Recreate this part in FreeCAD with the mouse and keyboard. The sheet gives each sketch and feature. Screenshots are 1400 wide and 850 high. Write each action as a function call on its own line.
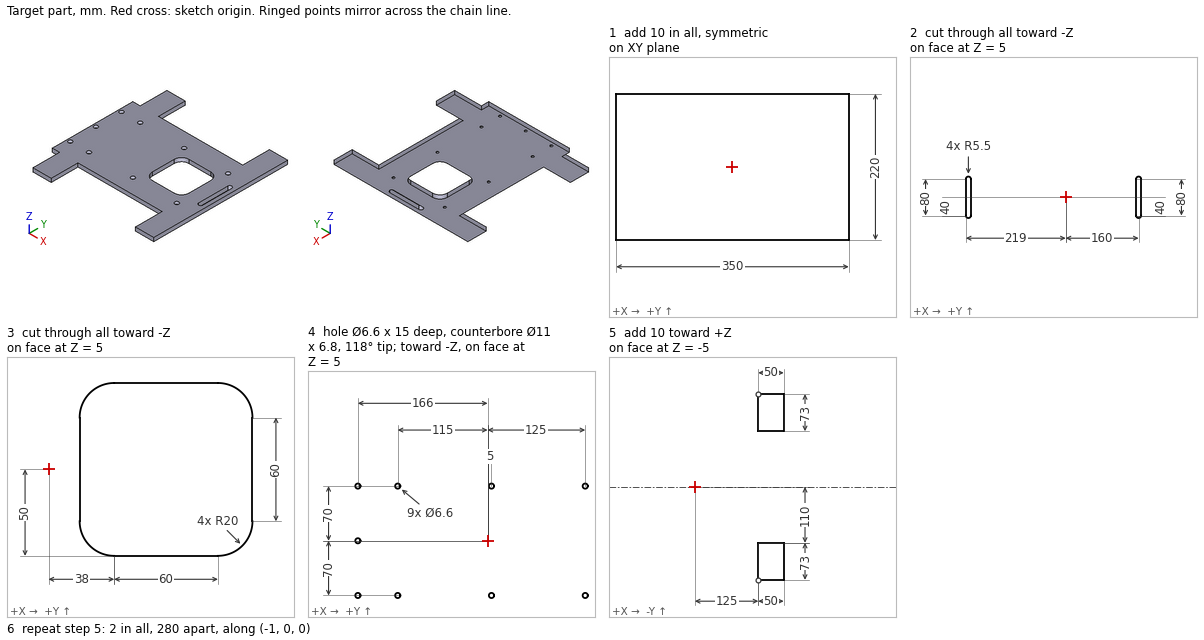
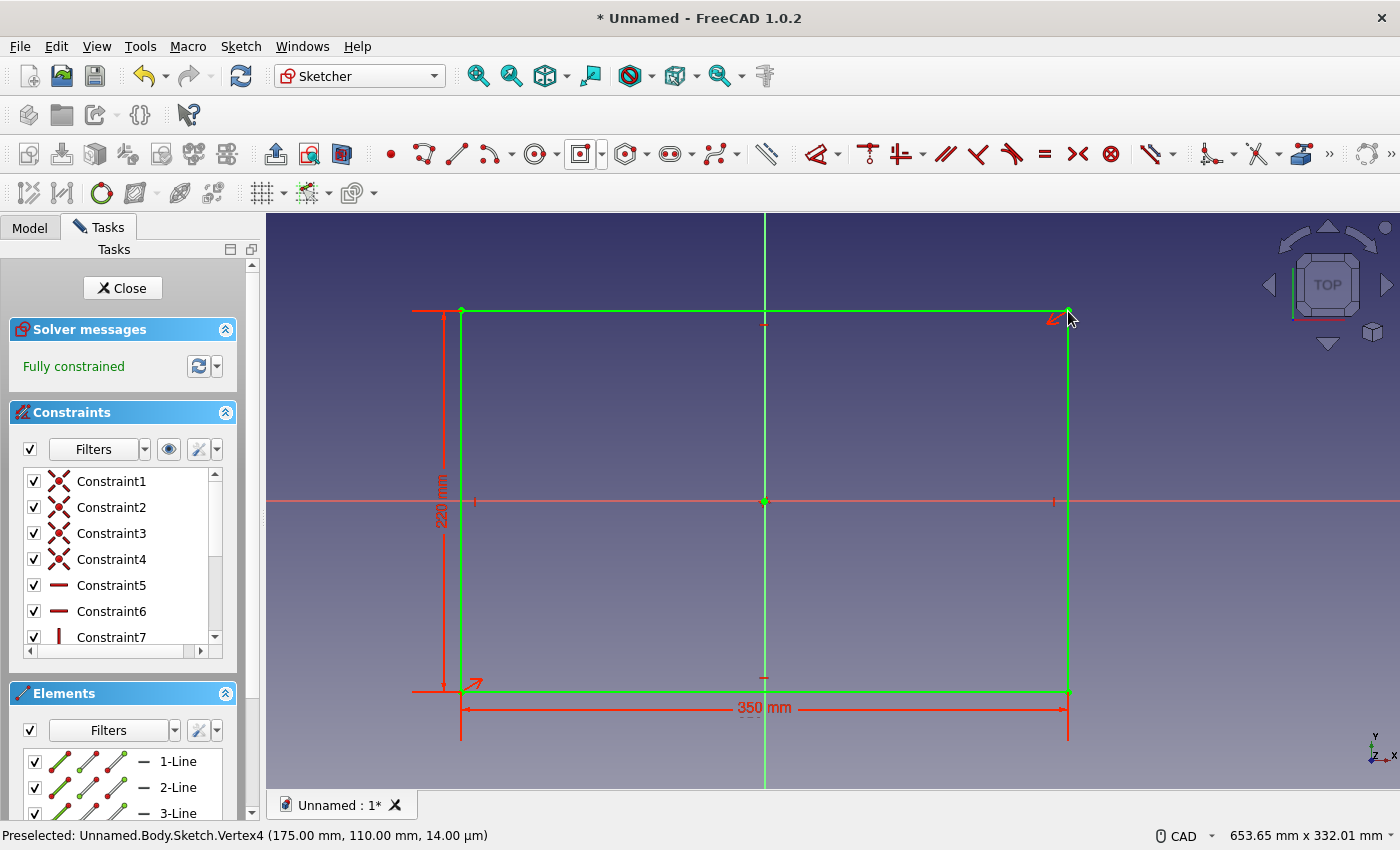
click(123, 288)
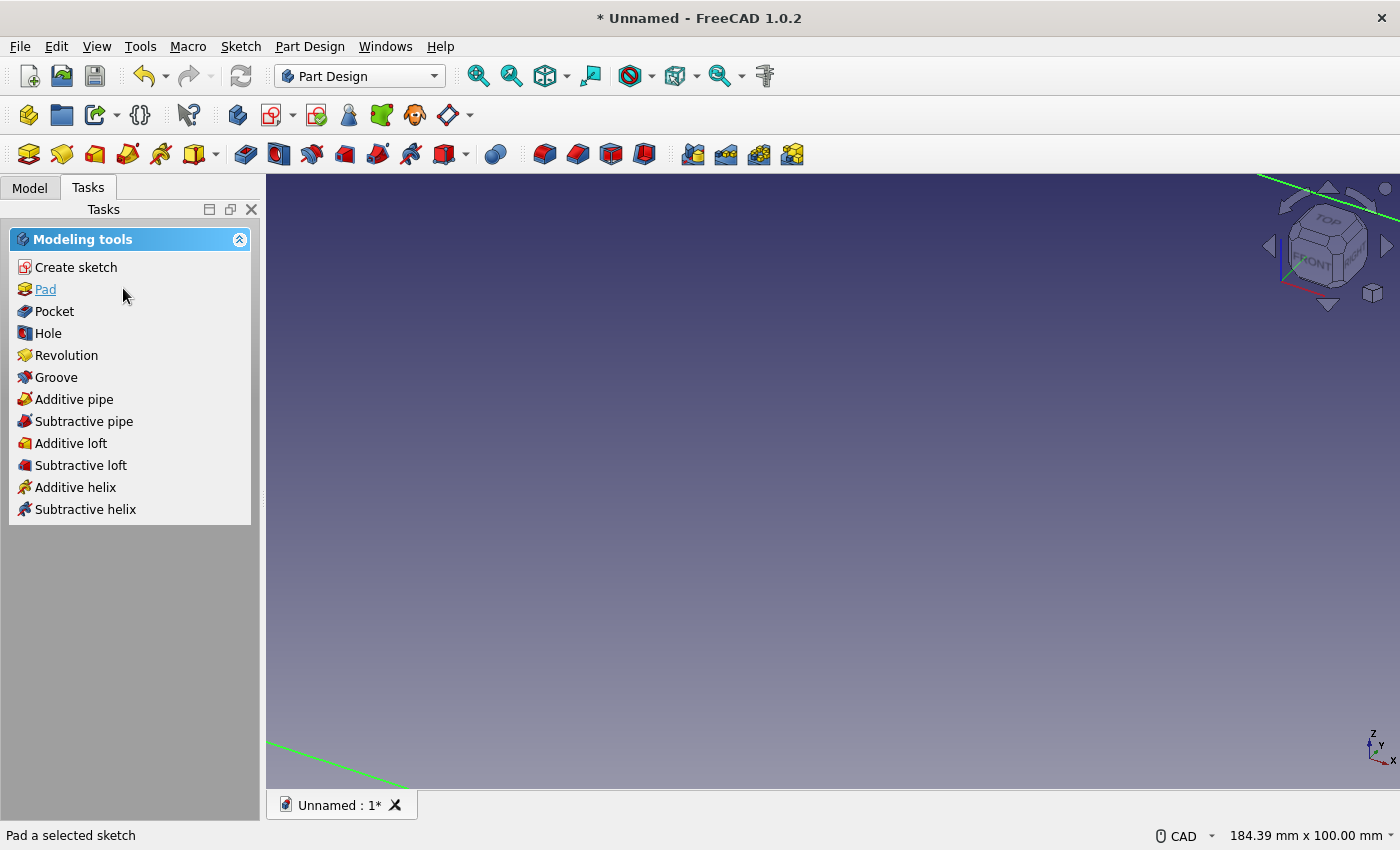
click(29, 154)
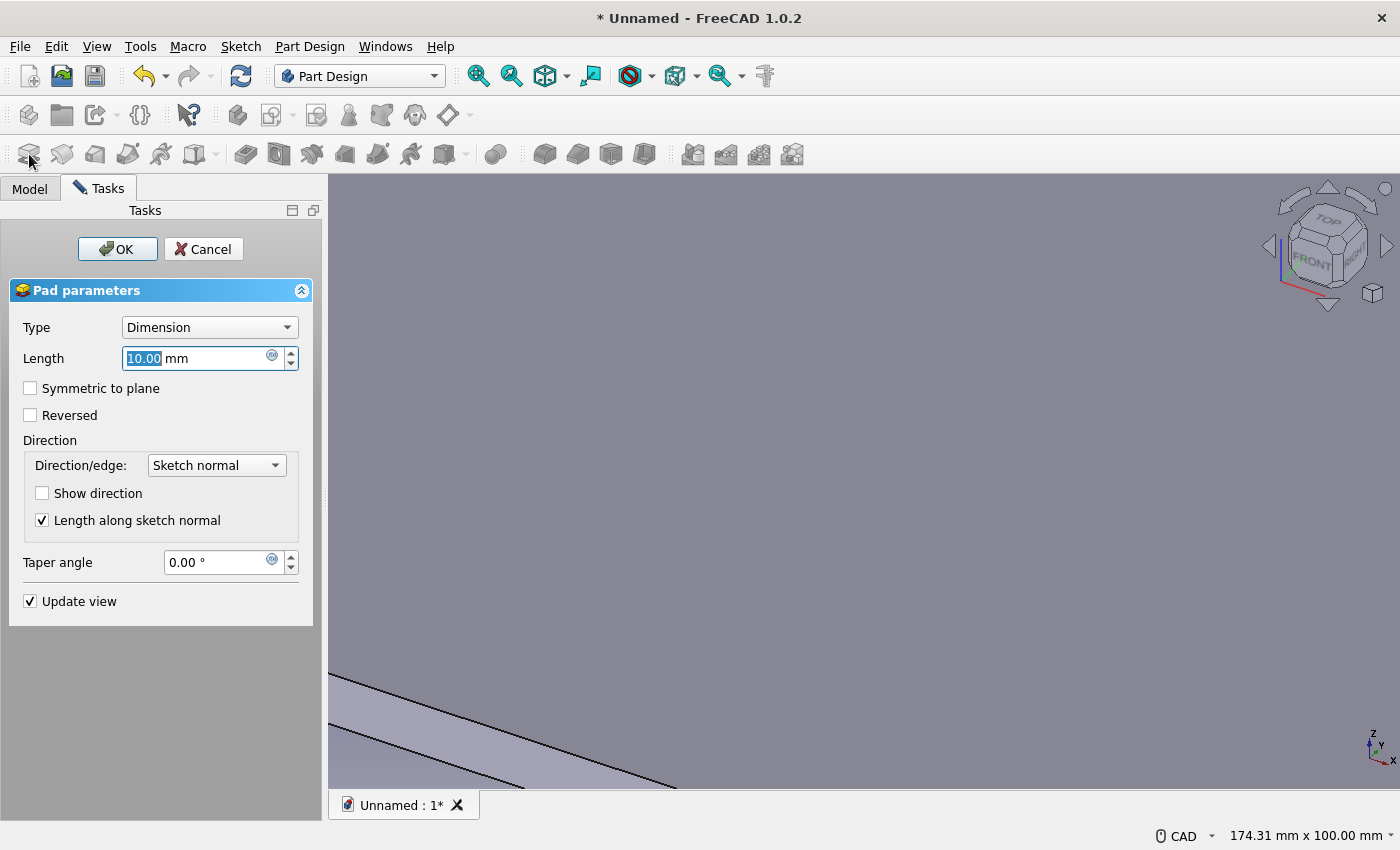
text(10)
key(Tab)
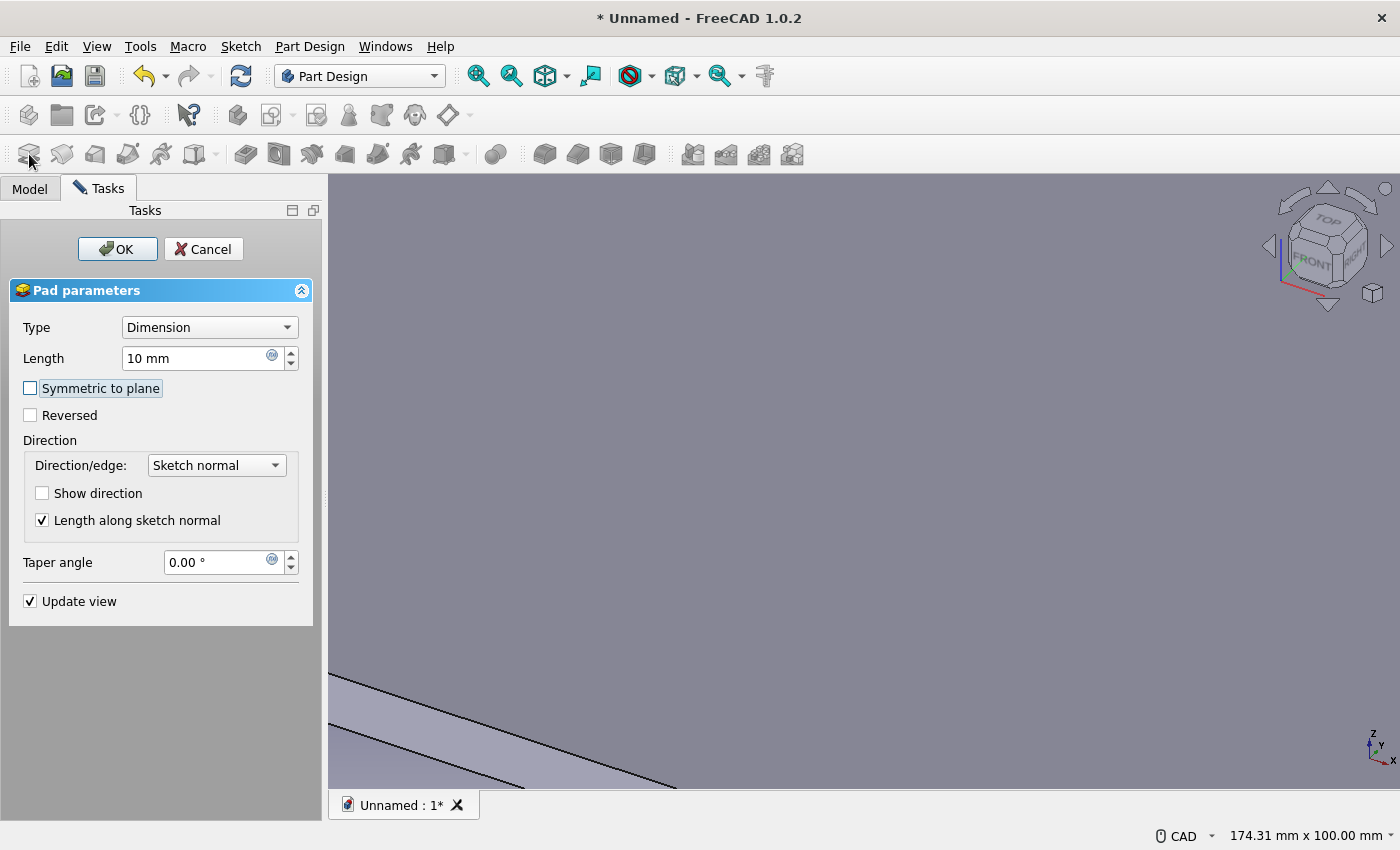
click(31, 388)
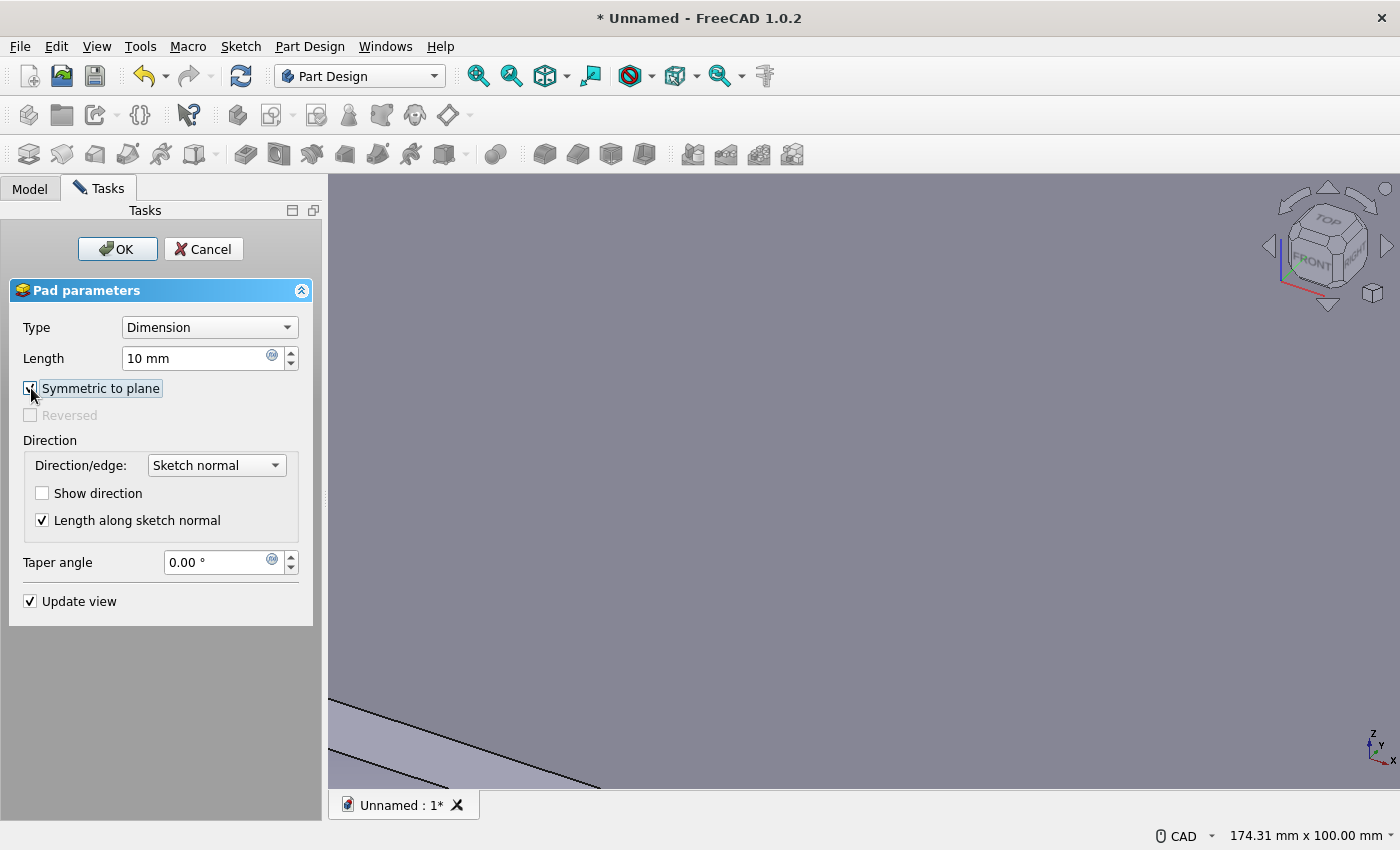
click(118, 249)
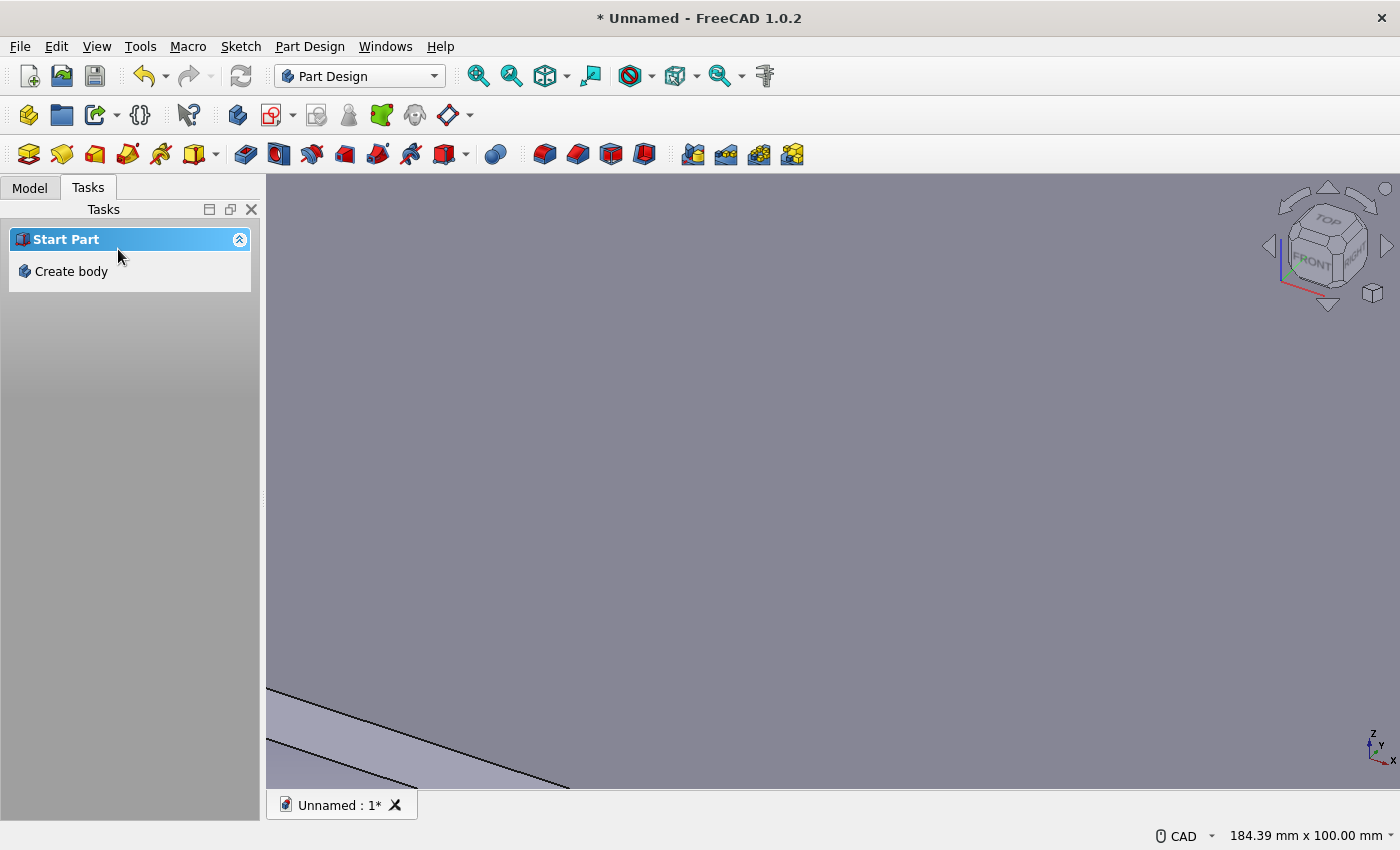
click(479, 76)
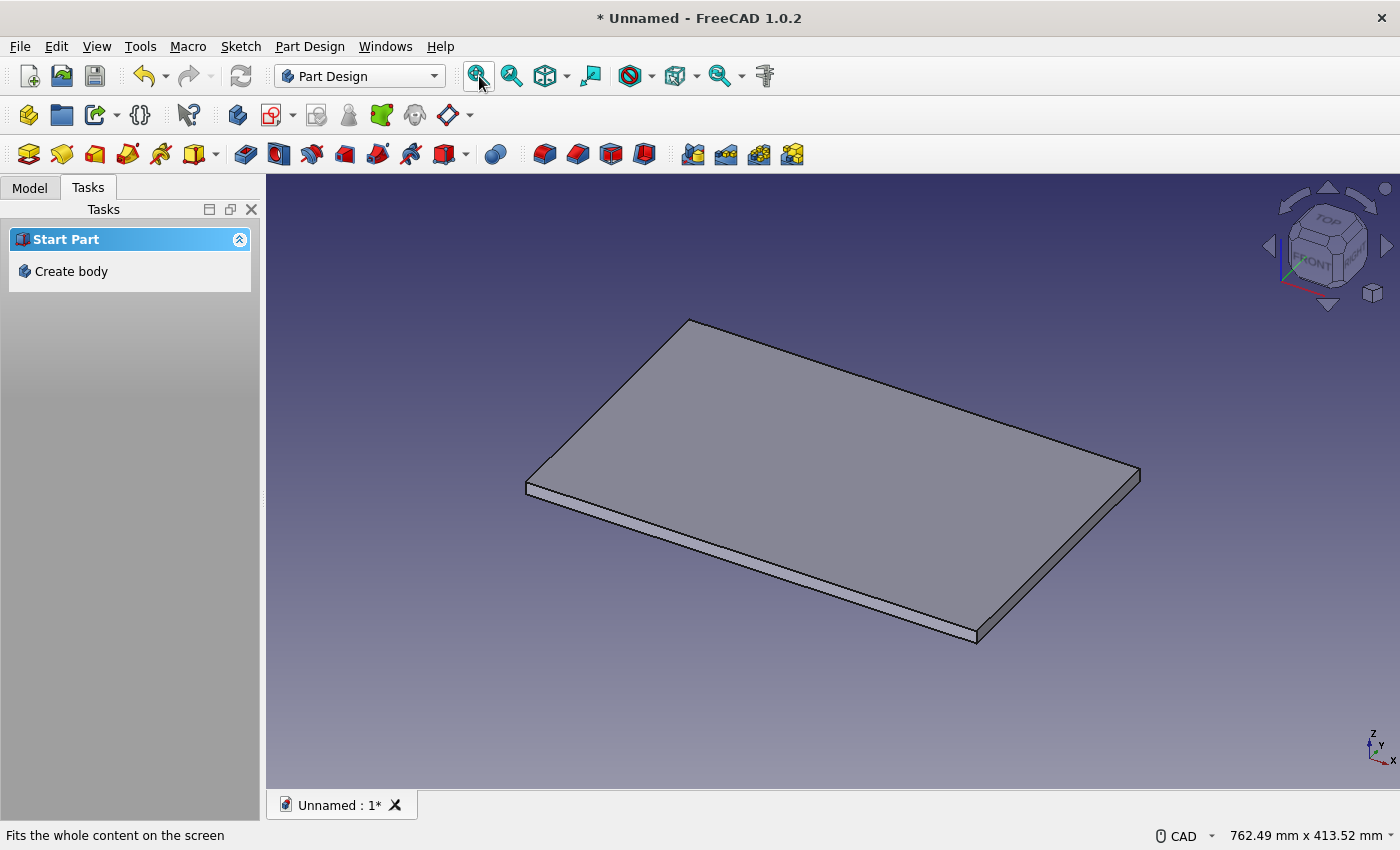
click(897, 496)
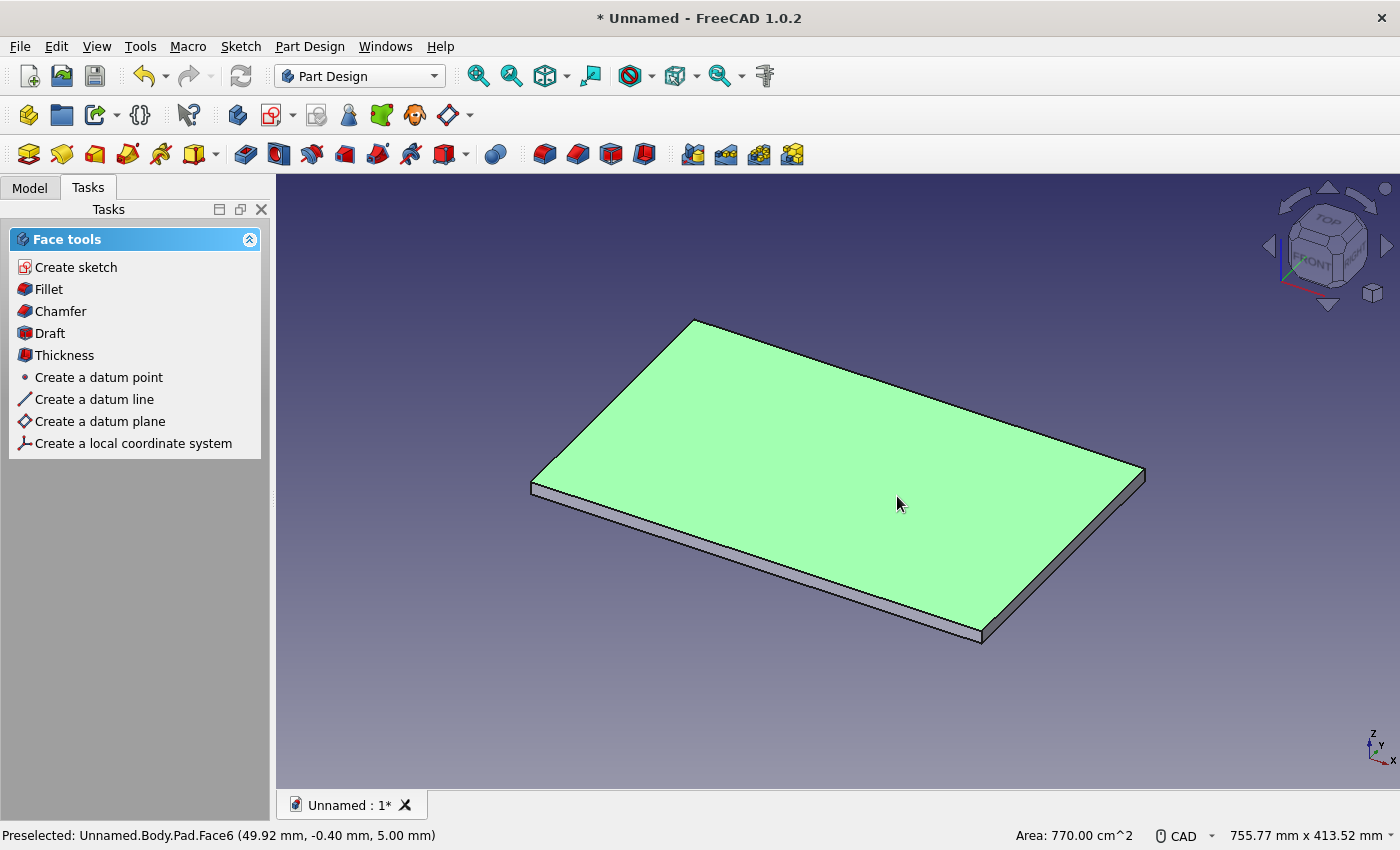
click(270, 116)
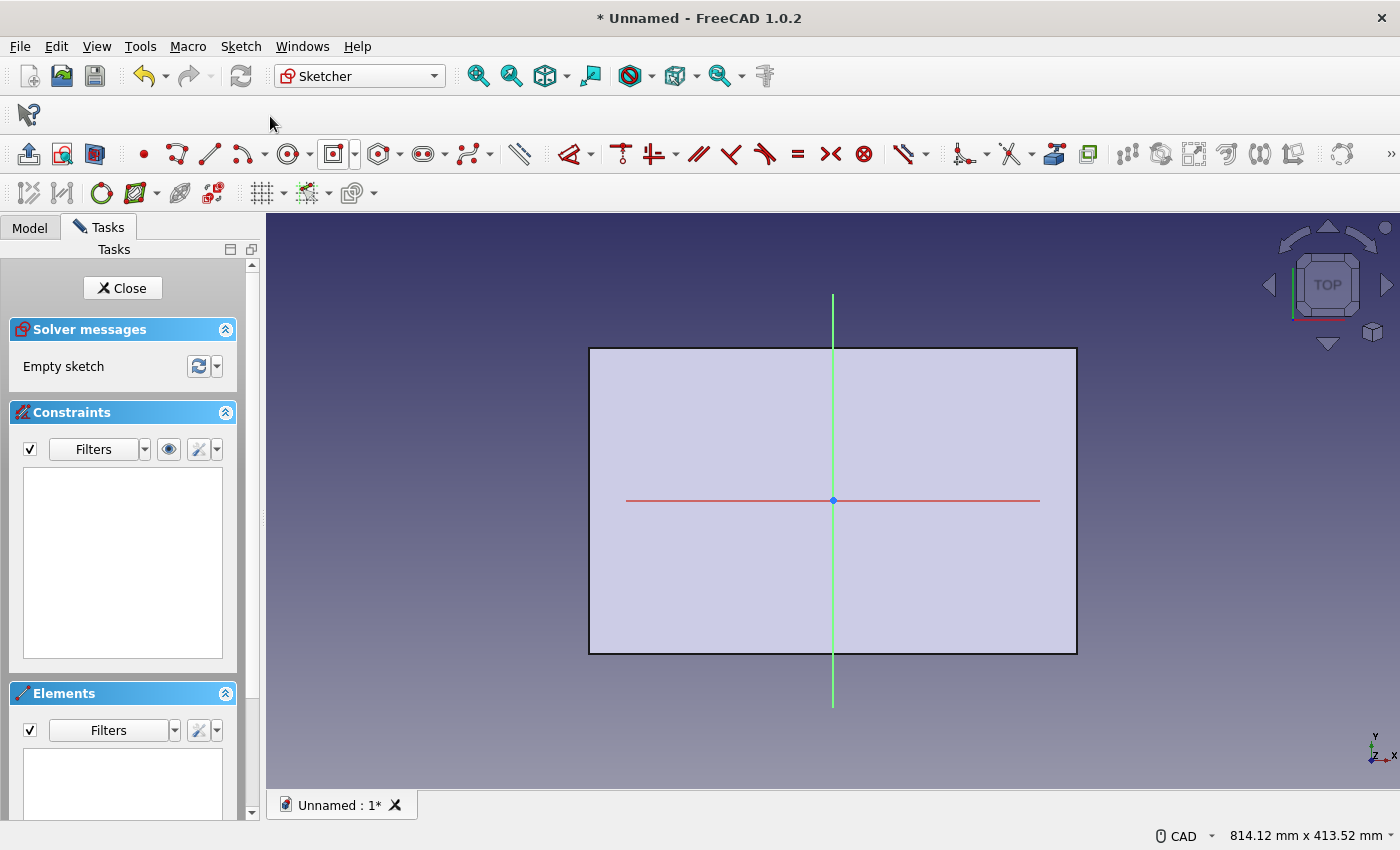
click(422, 154)